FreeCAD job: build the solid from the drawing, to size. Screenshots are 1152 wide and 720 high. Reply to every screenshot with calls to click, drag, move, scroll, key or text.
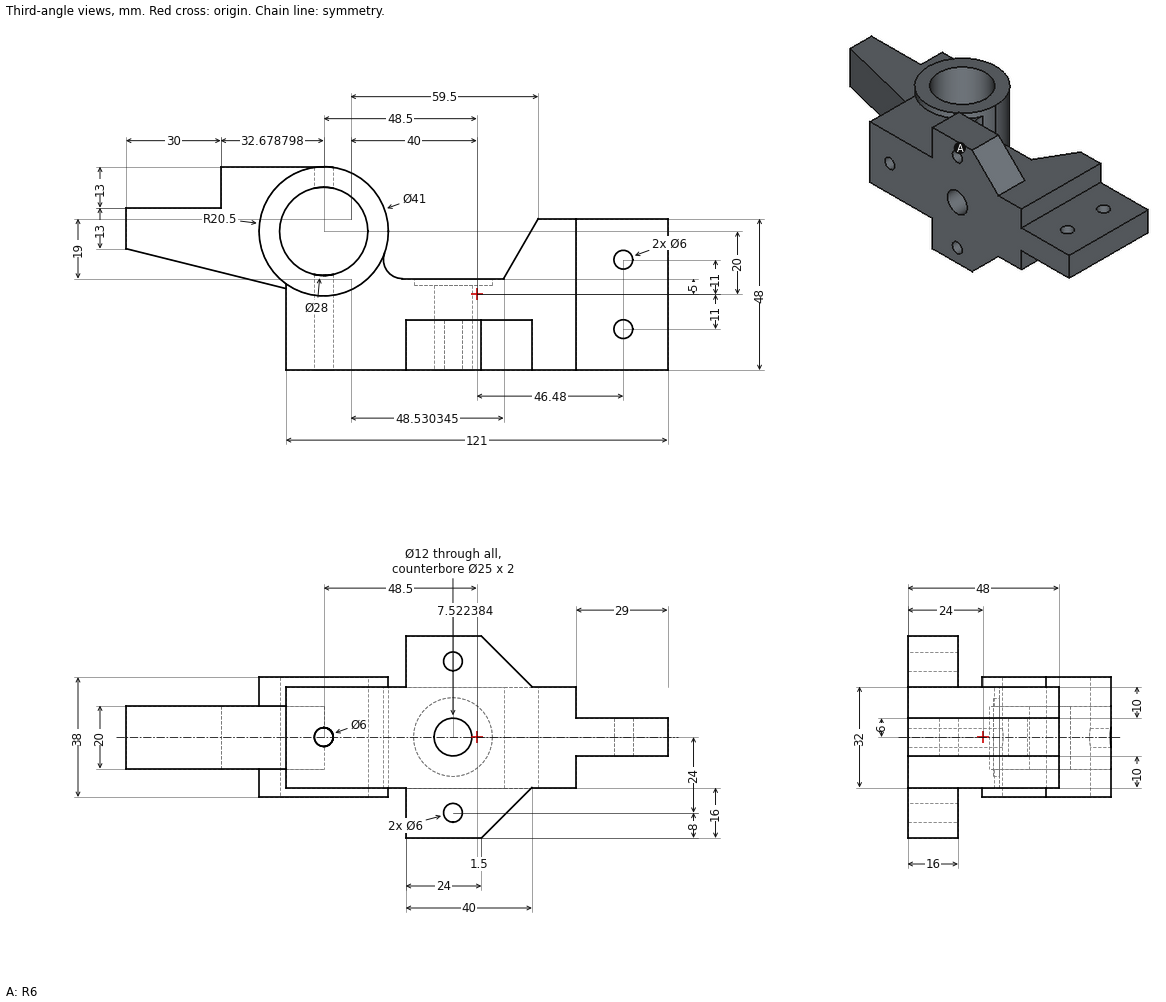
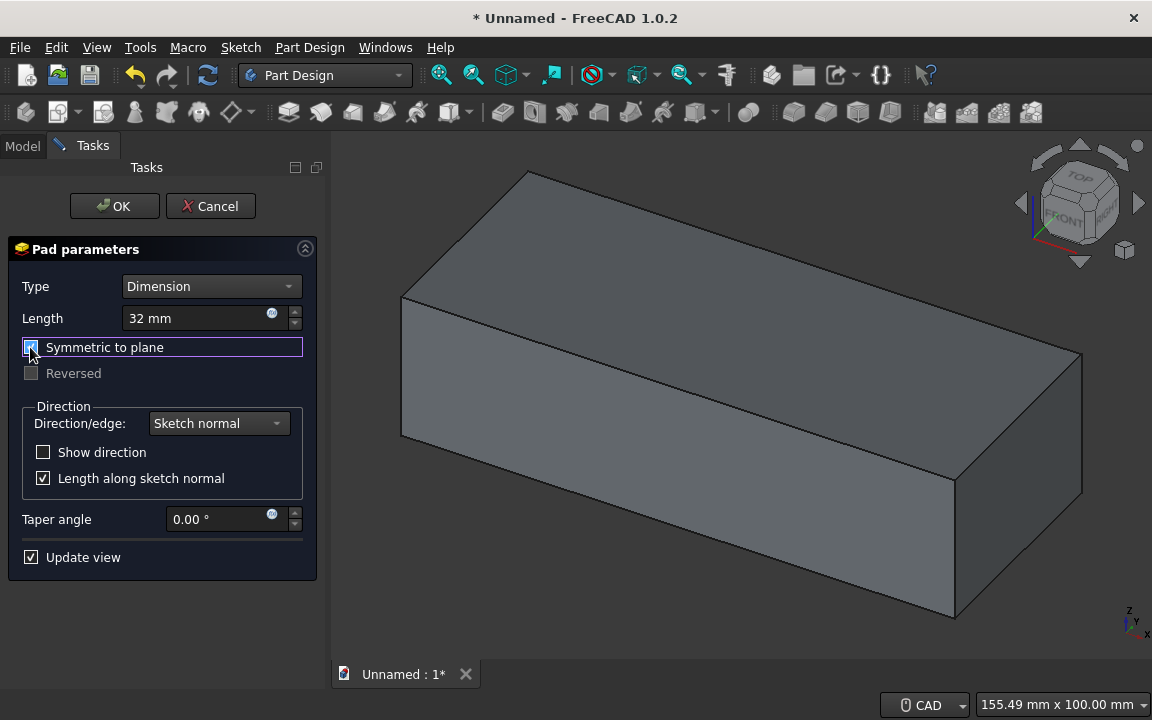
click(115, 206)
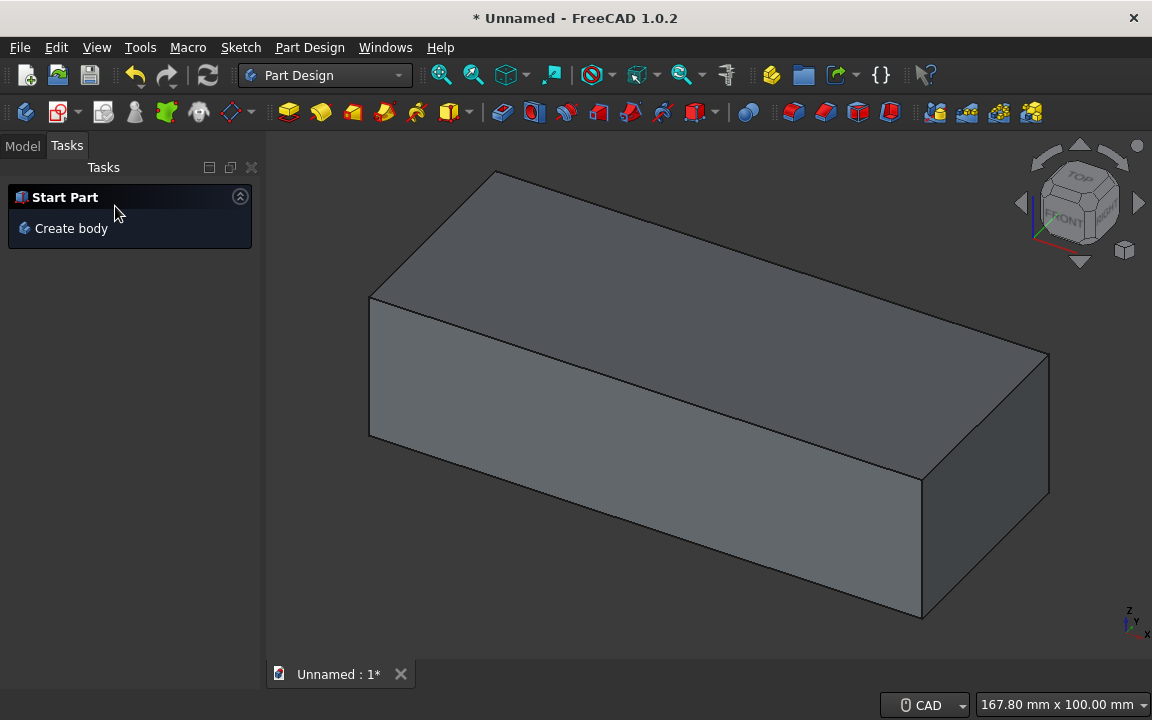
click(1004, 468)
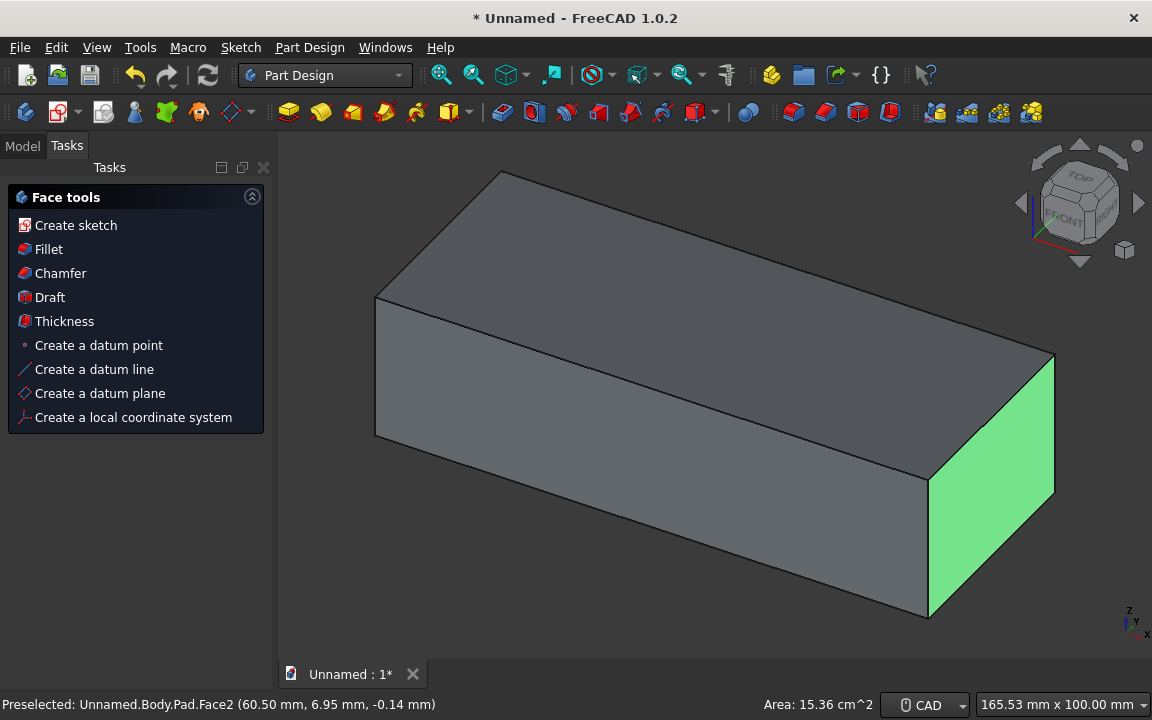
click(58, 112)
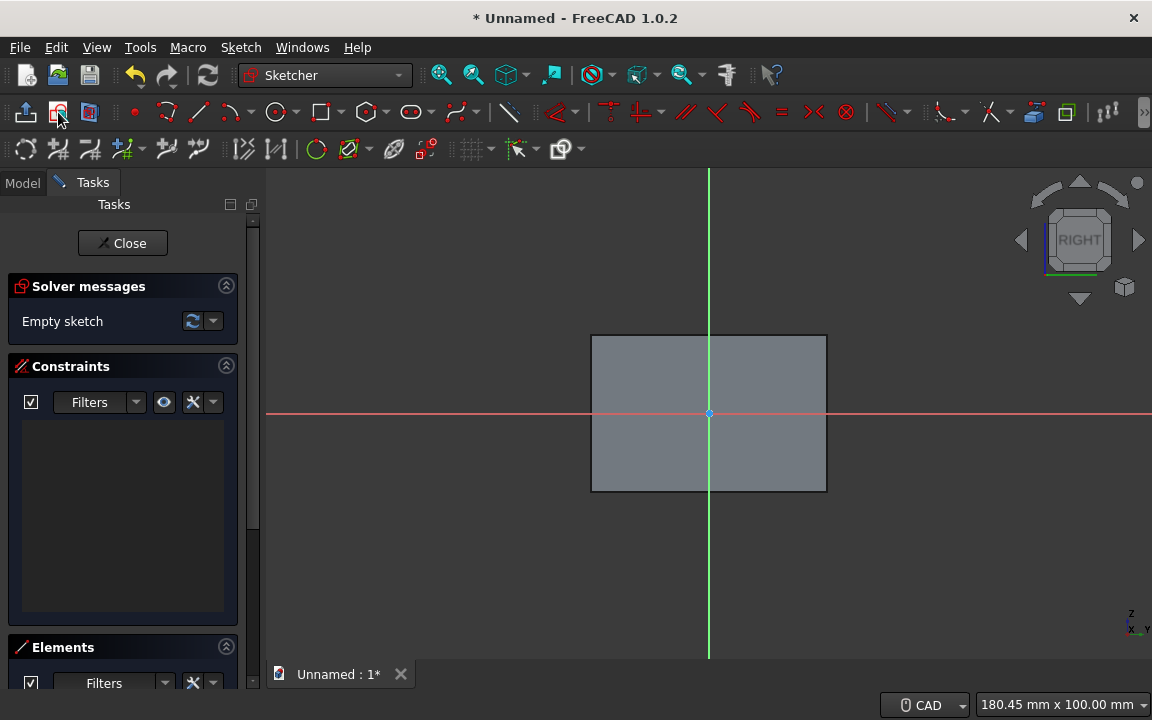
scroll(792, 414, up, 3)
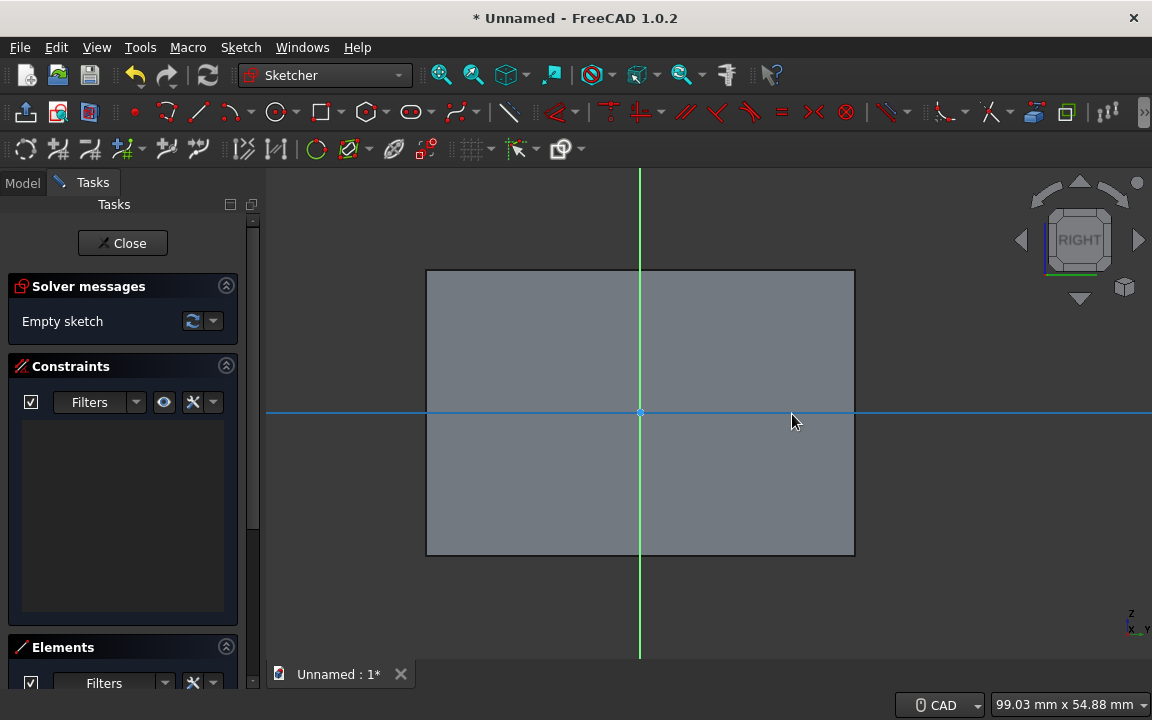
key(g)
key(r)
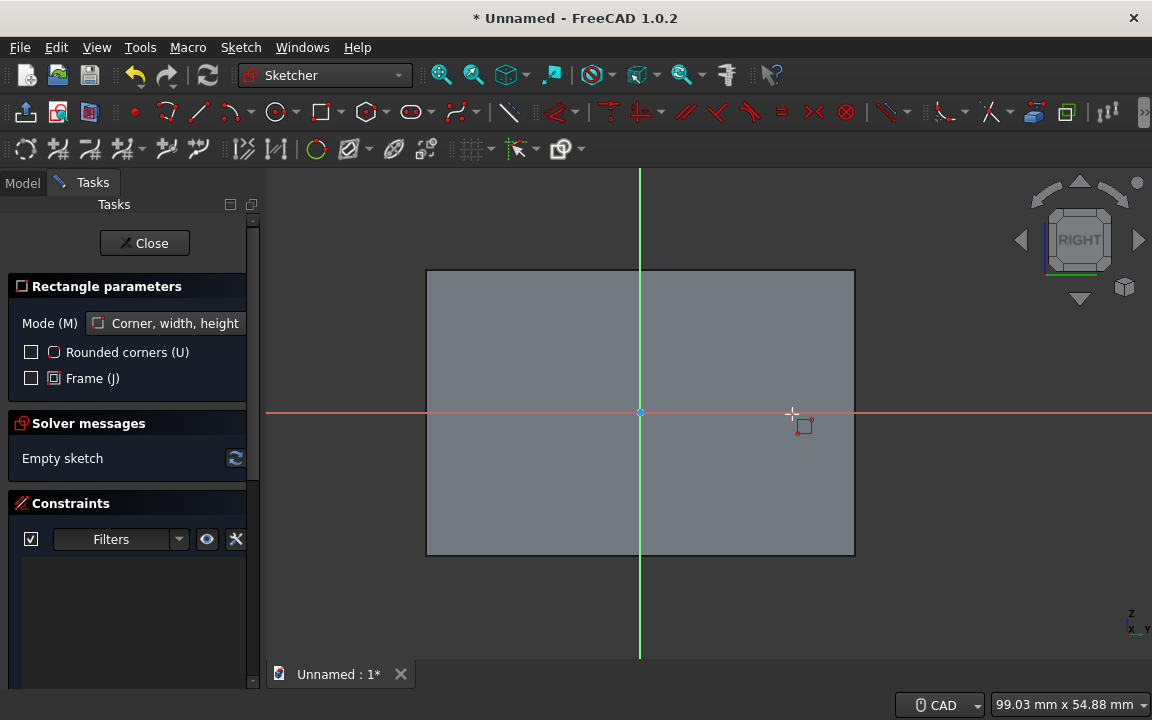
click(426, 270)
move(855, 359)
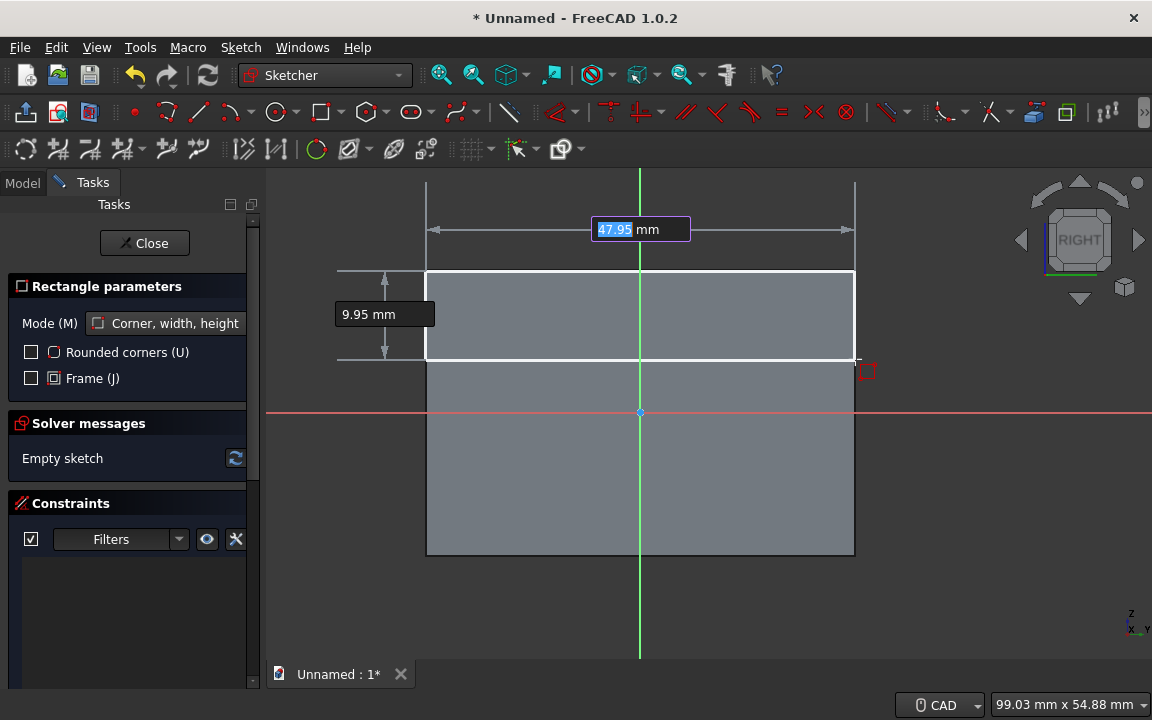
text(48)
key(Tab)
text(10)
key(Return)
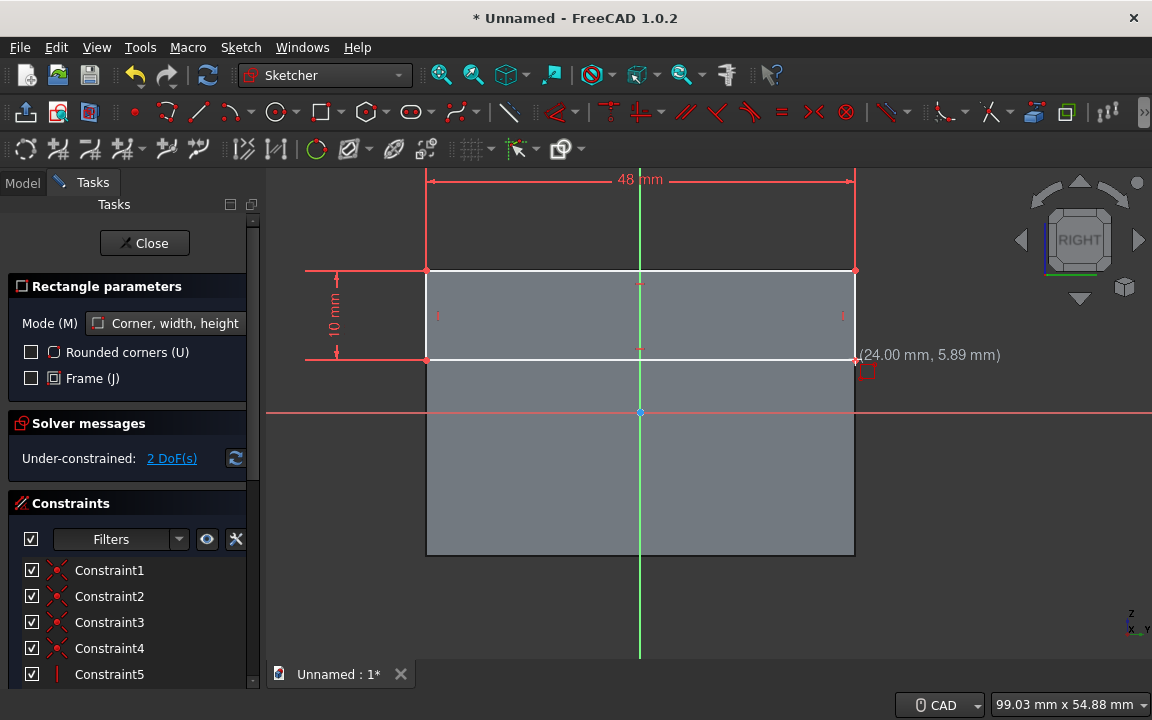
click(426, 466)
move(855, 556)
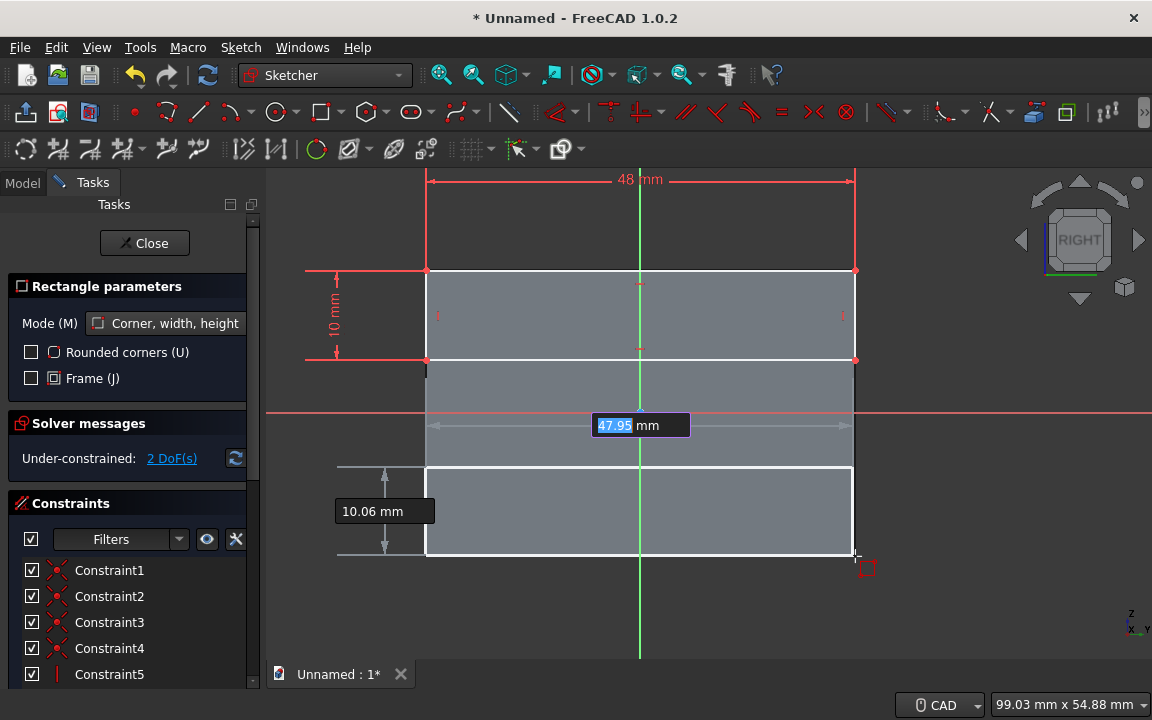
text(48)
key(Tab)
text(10)
key(Return)
key(Escape)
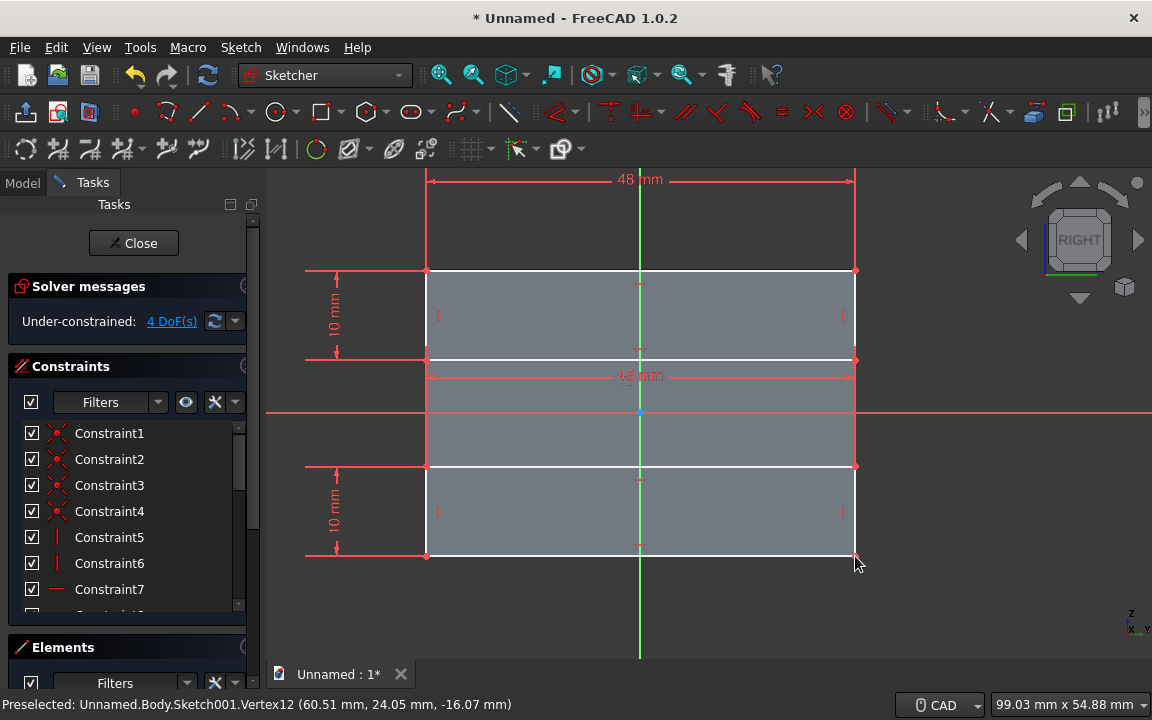
click(426, 360)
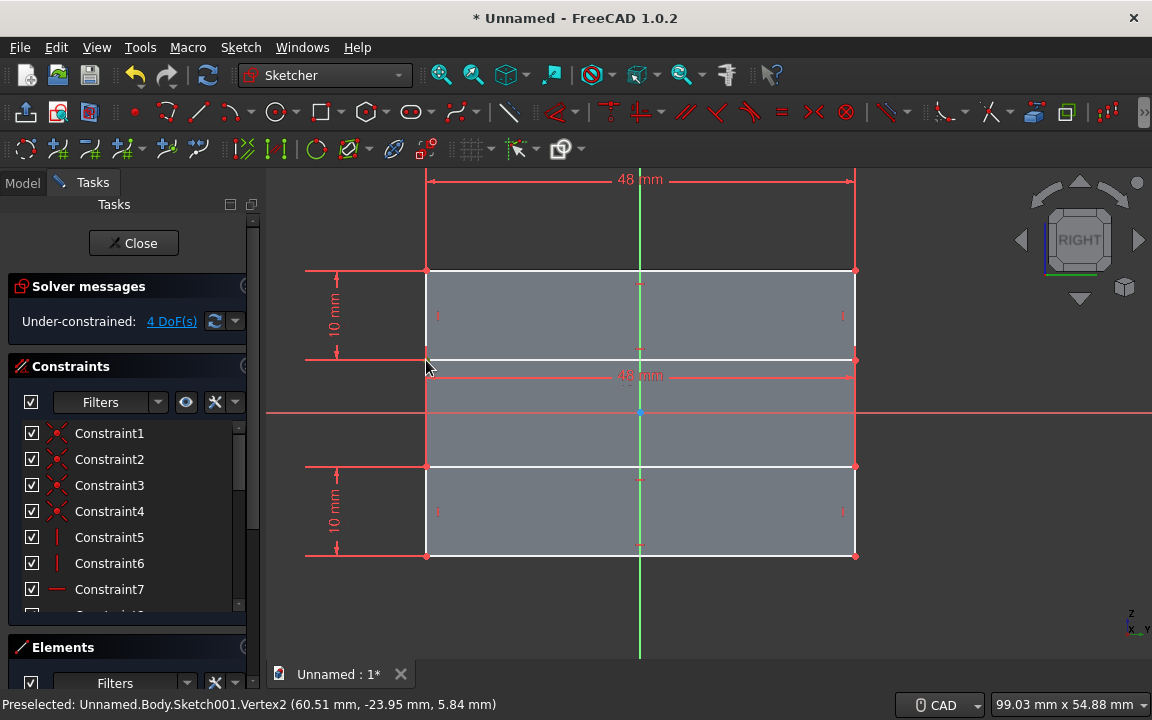
click(426, 467)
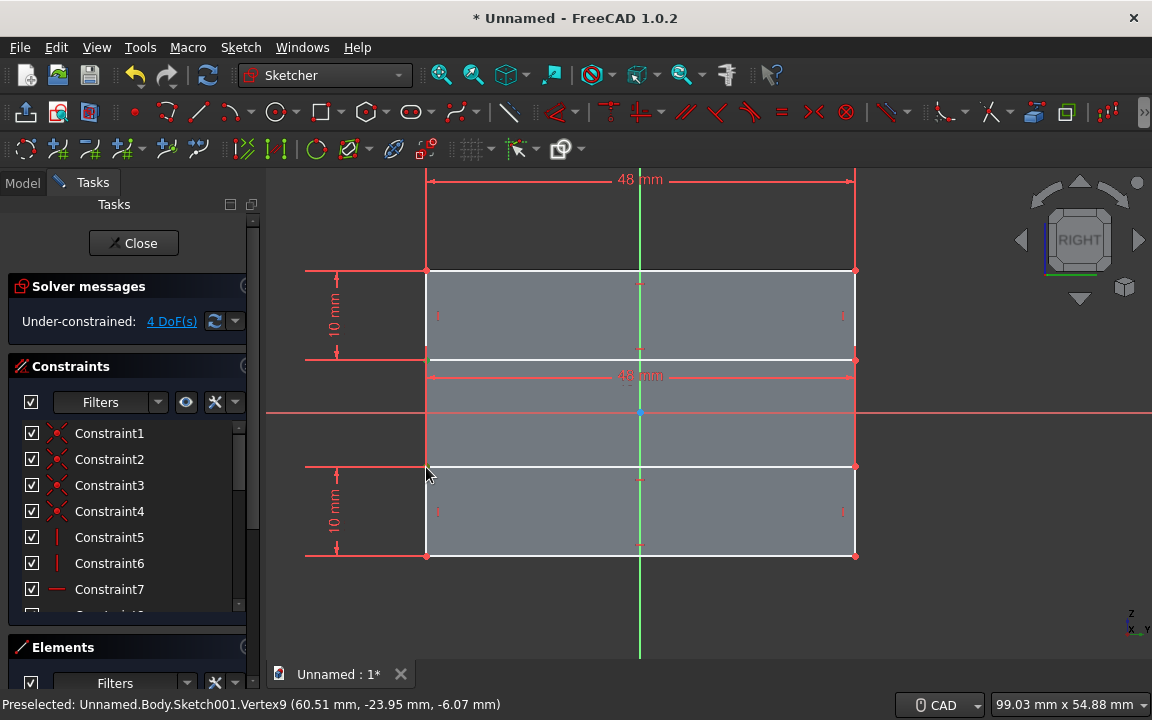
click(344, 413)